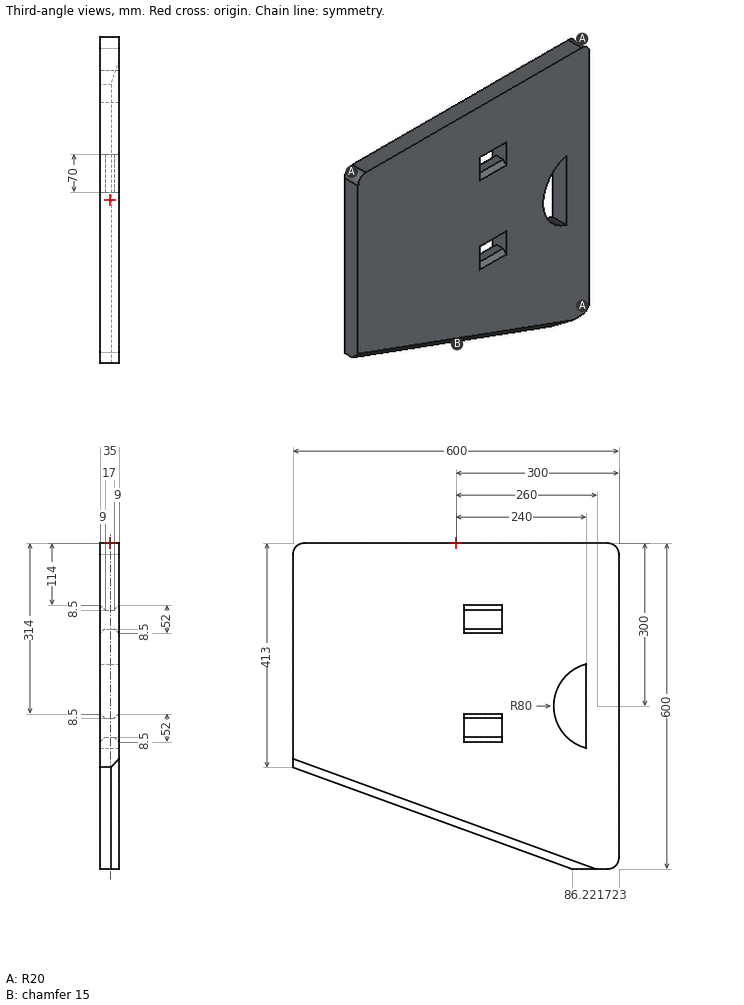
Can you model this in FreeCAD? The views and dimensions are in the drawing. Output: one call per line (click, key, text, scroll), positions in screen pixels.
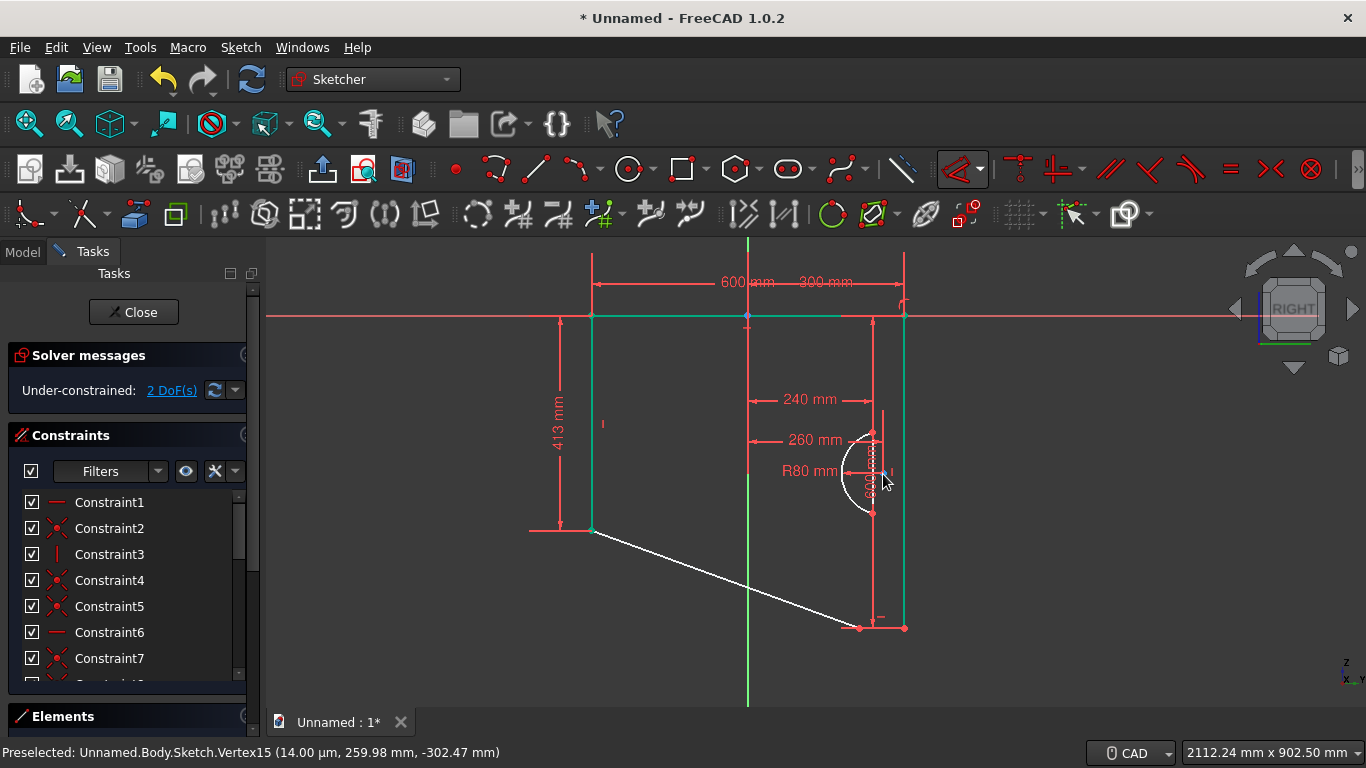
click(883, 473)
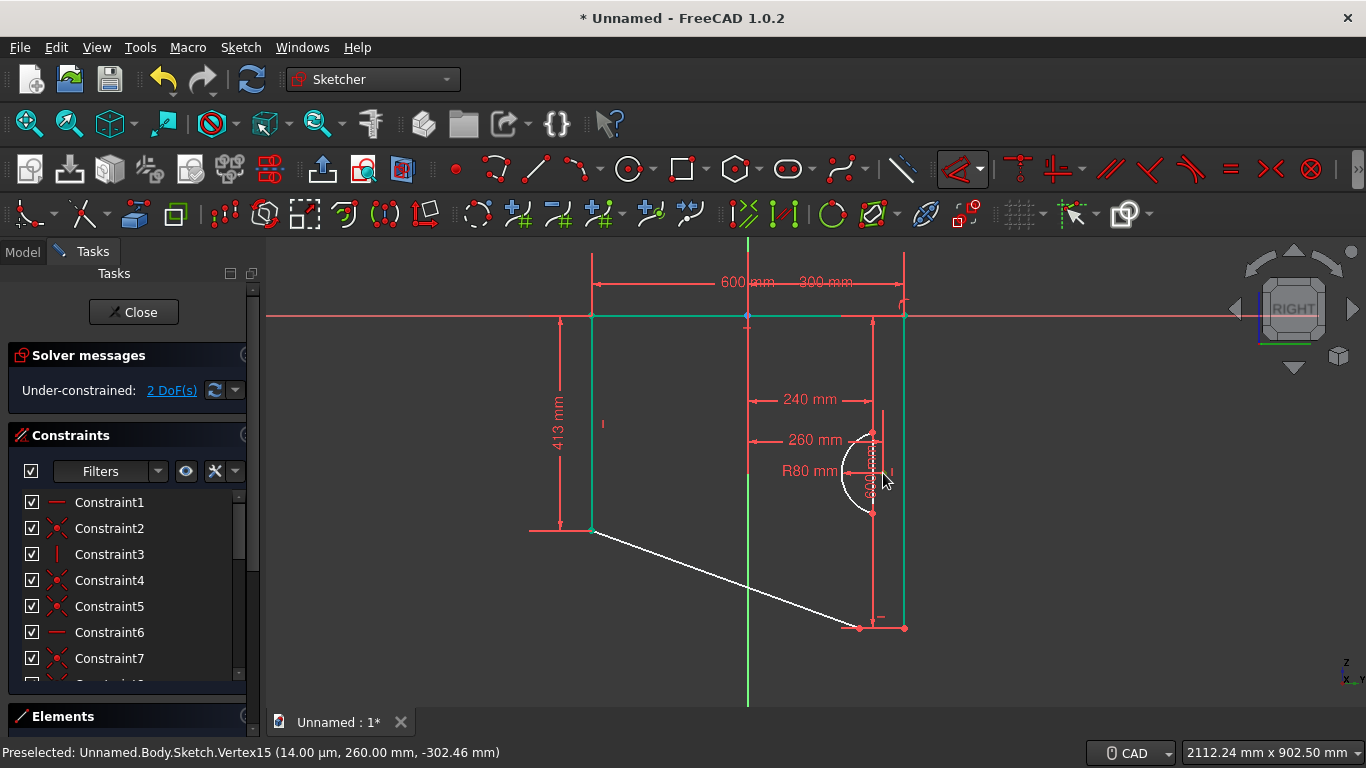
key(i)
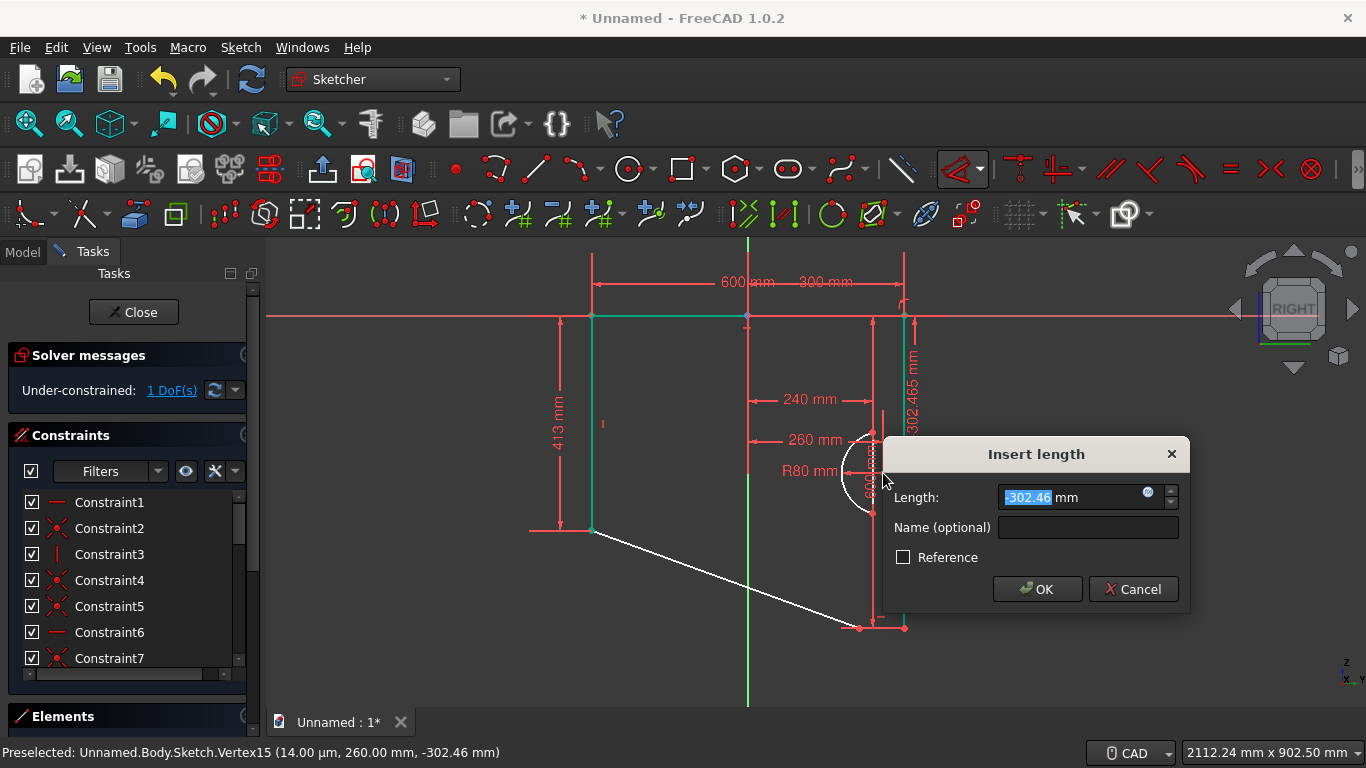
text(-300)
key(Return)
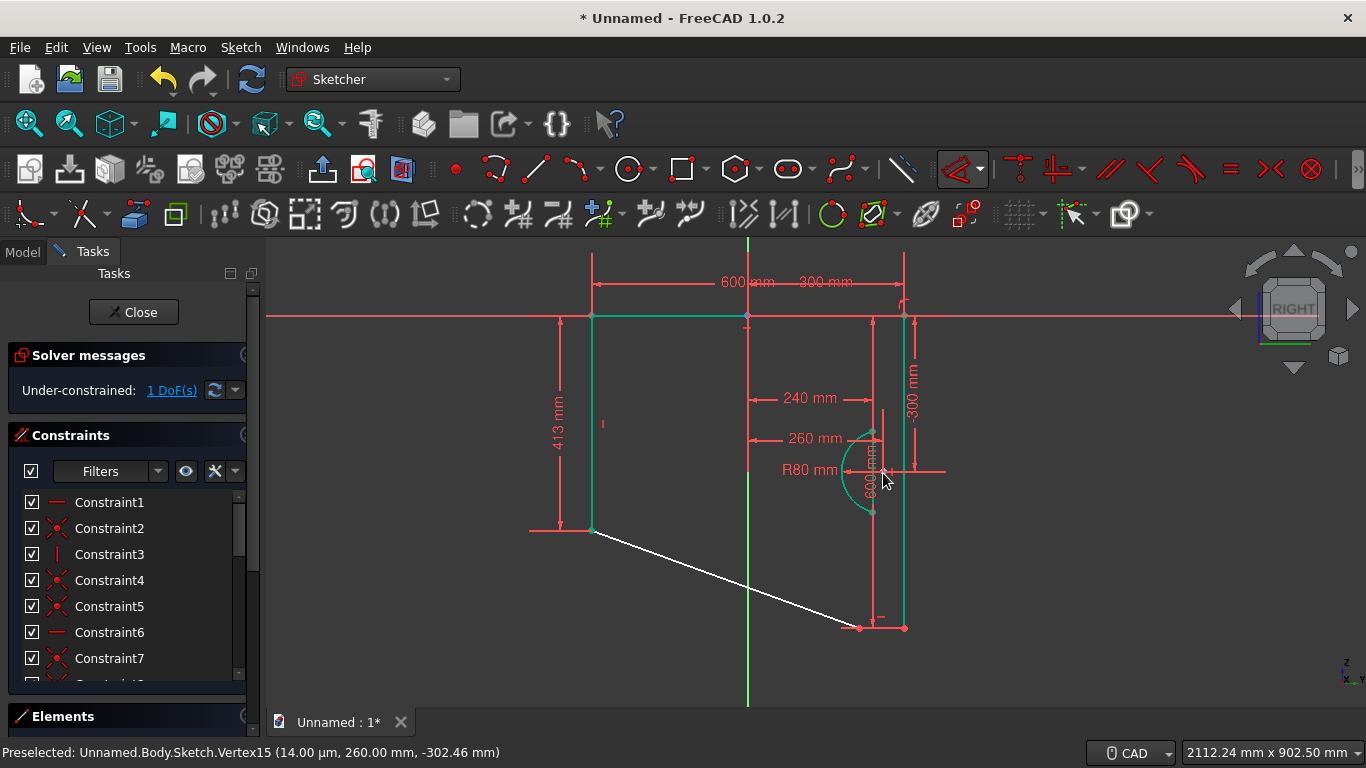
click(873, 628)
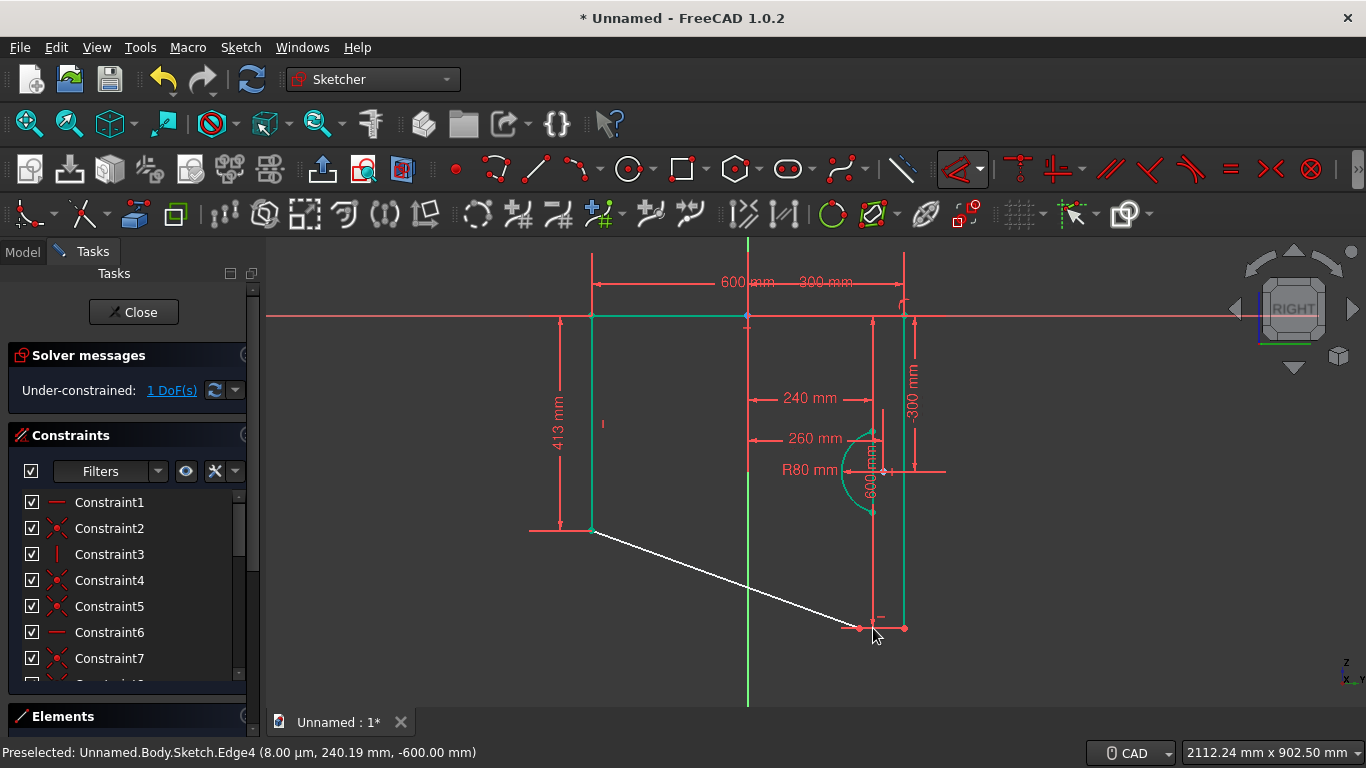
key(l)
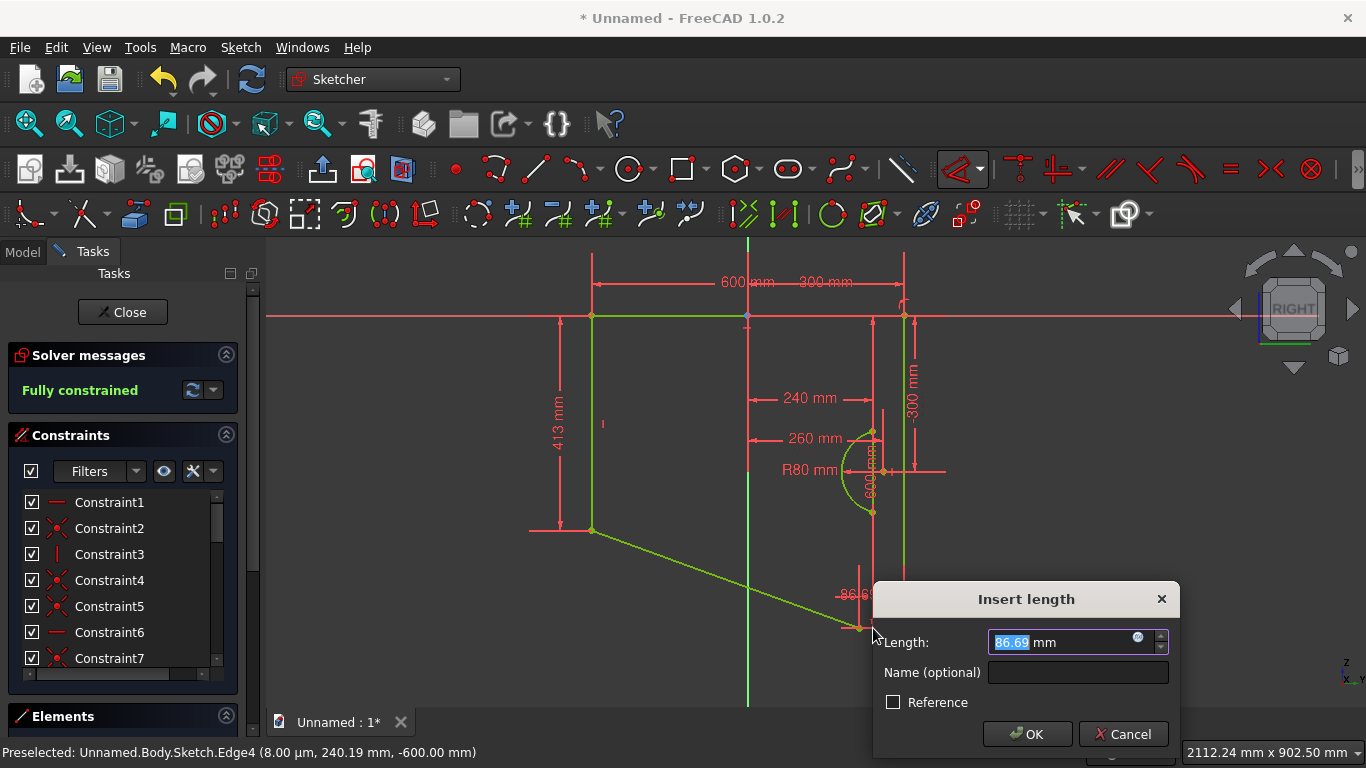
text(86.221723)
key(Return)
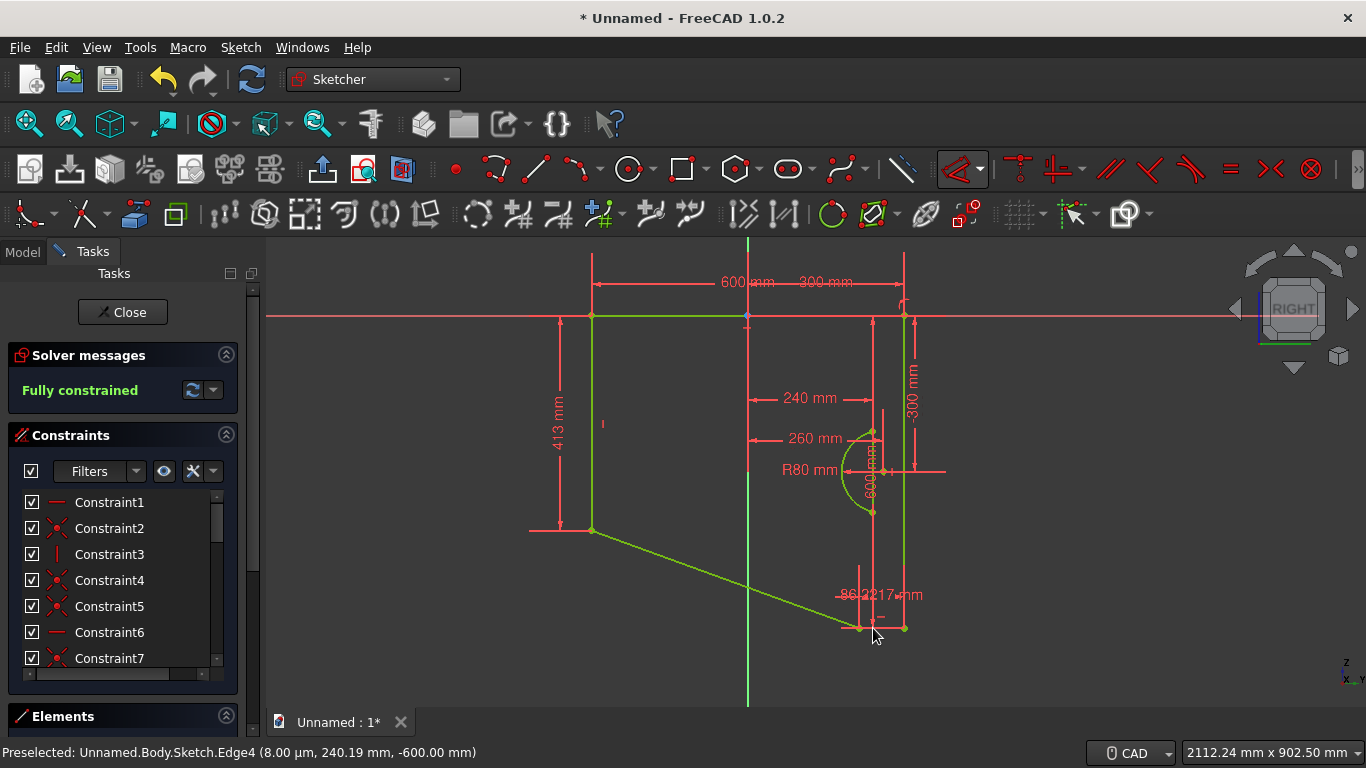
click(123, 312)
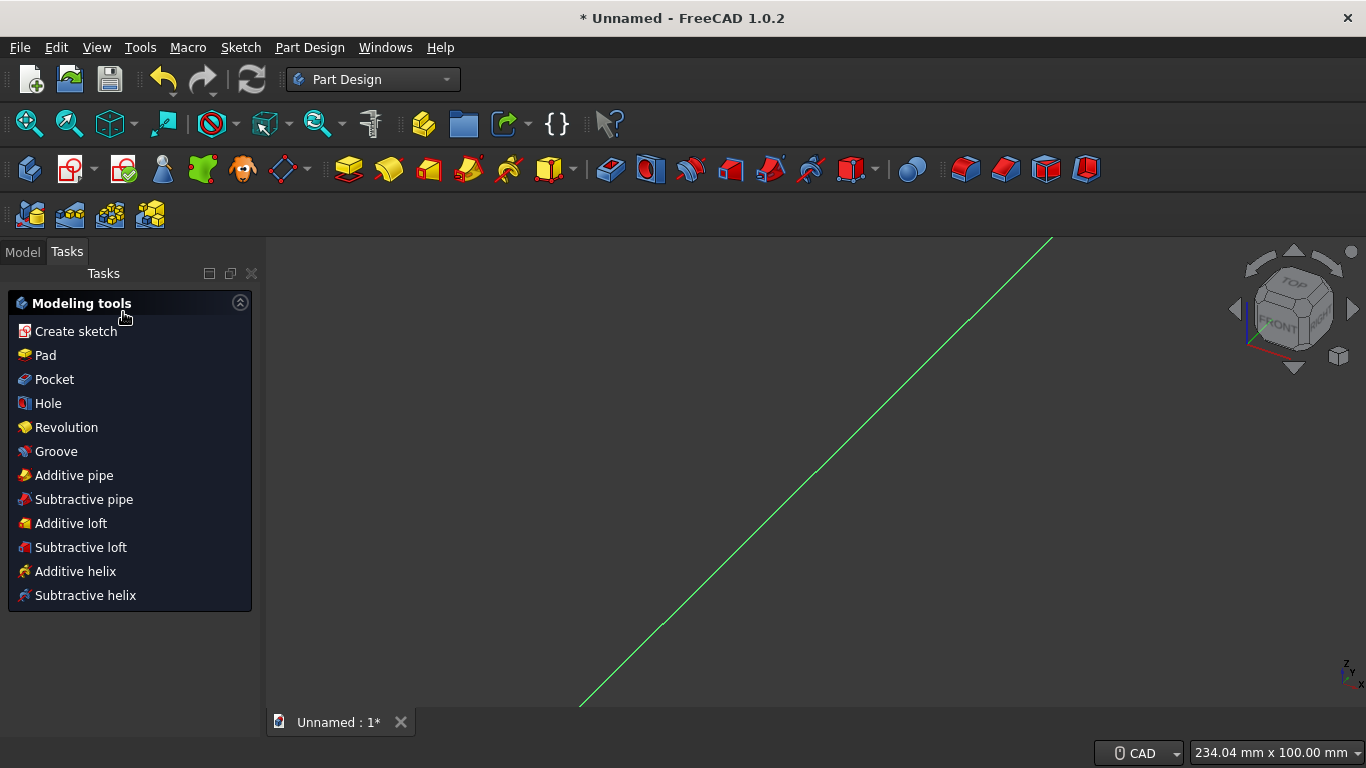
click(350, 170)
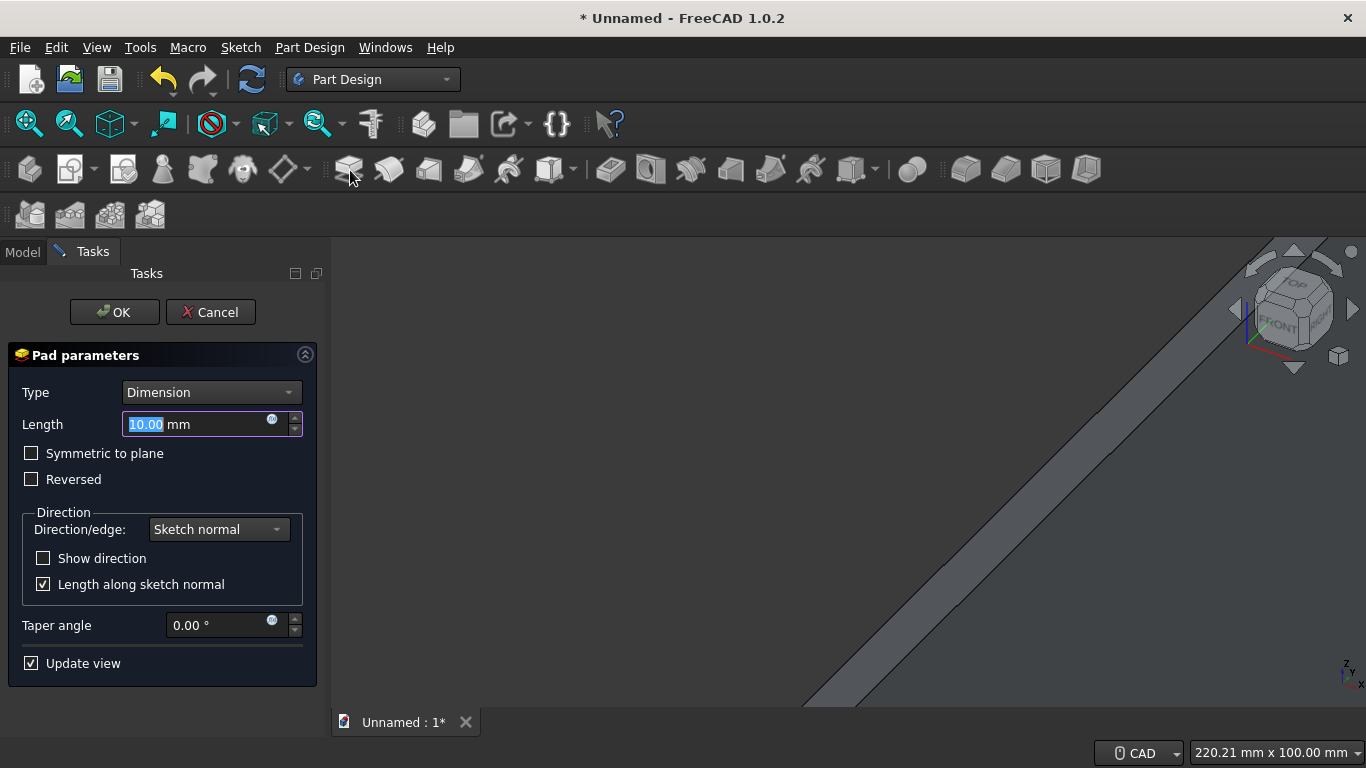
text(35)
key(Tab)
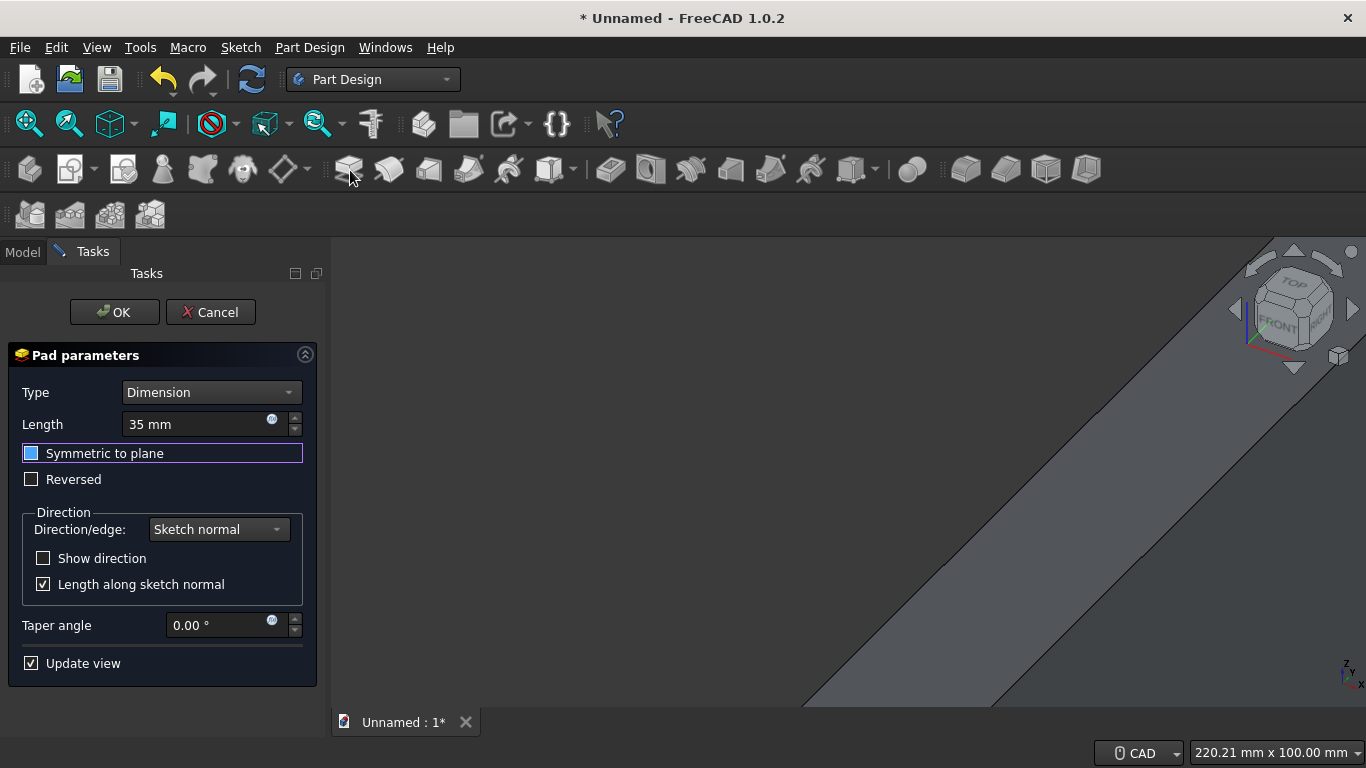
click(30, 453)